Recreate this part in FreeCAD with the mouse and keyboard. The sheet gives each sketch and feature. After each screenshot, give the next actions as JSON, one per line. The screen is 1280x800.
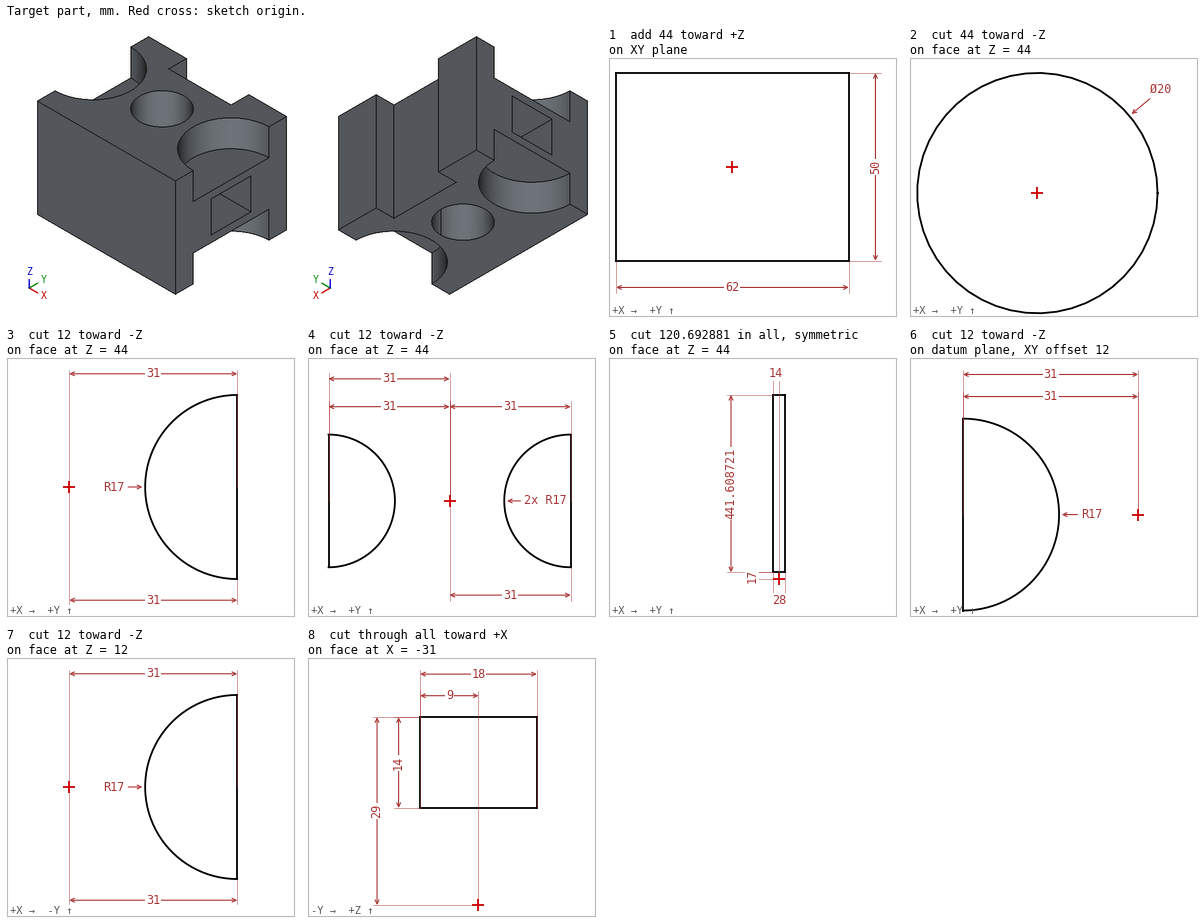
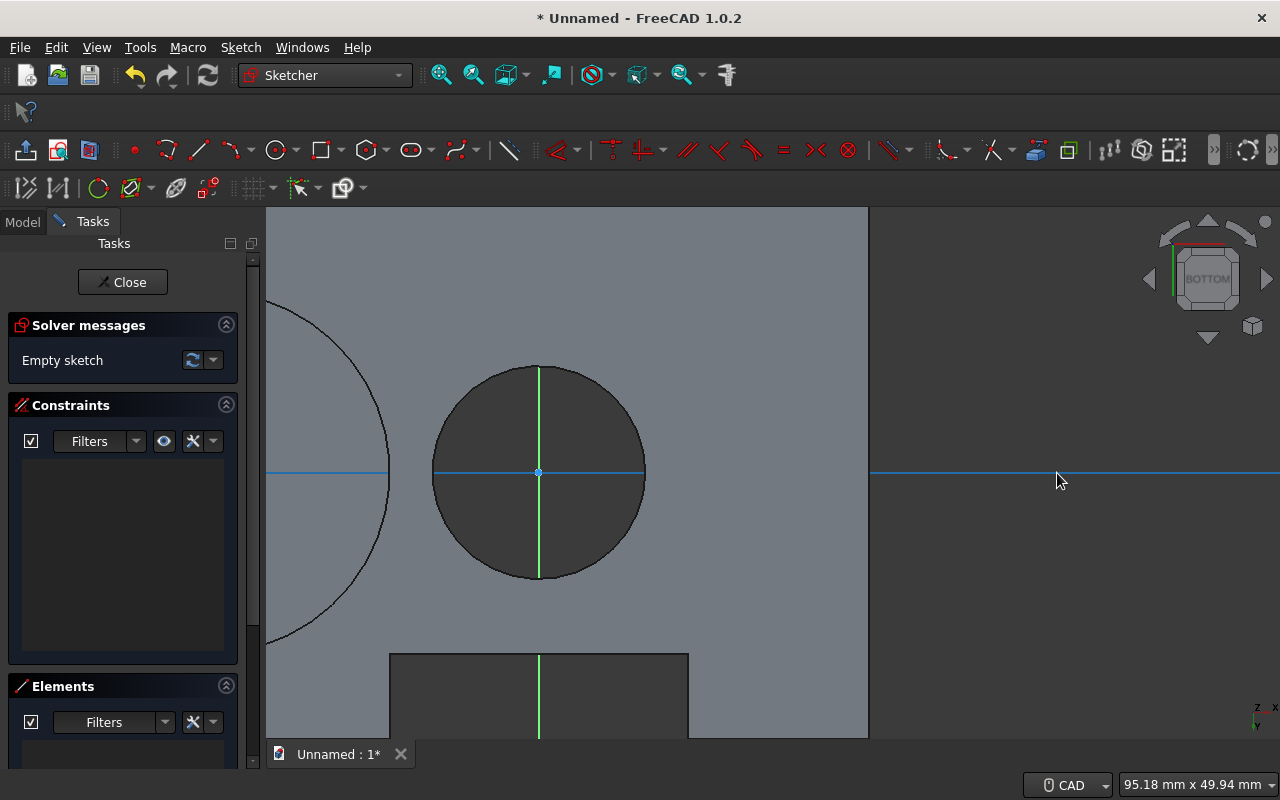
{"action": "left_click", "coordinate": [200, 150]}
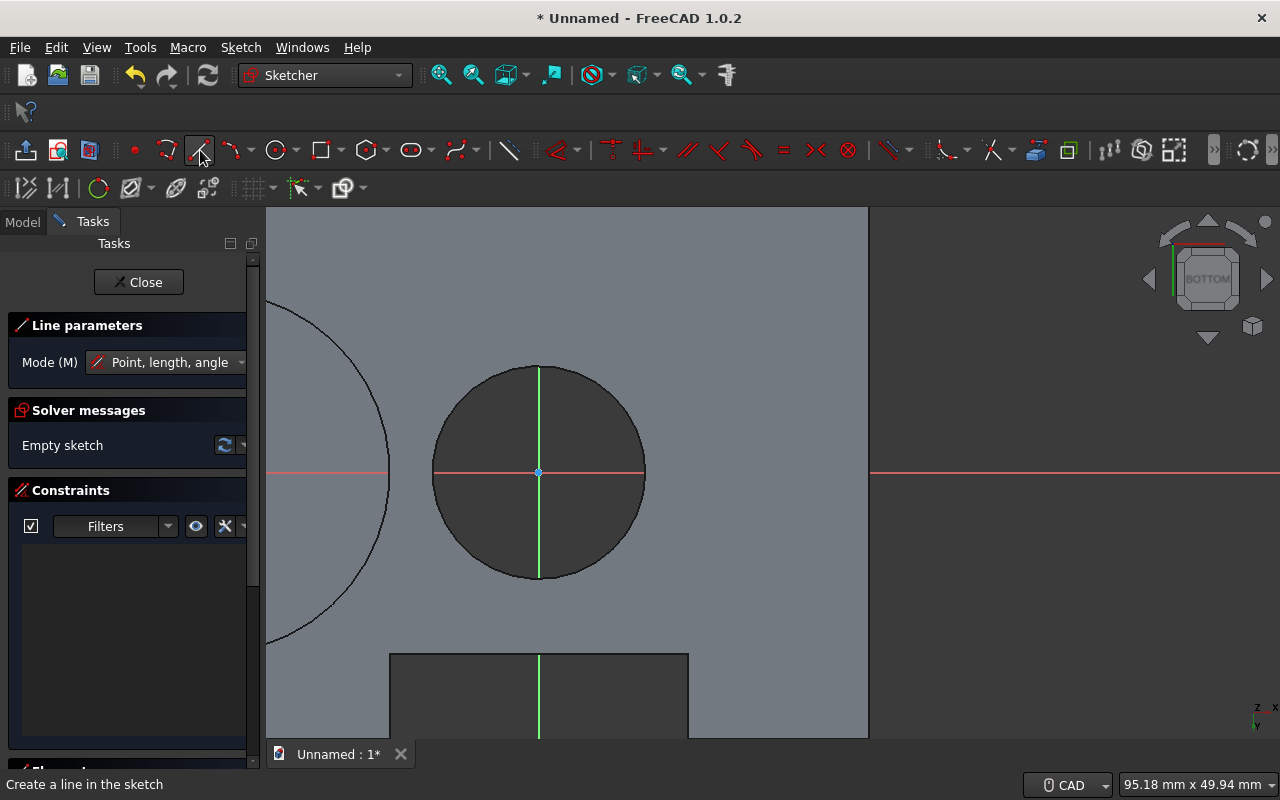
{"action": "left_click", "coordinate": [869, 654]}
{"action": "left_click", "coordinate": [869, 291]}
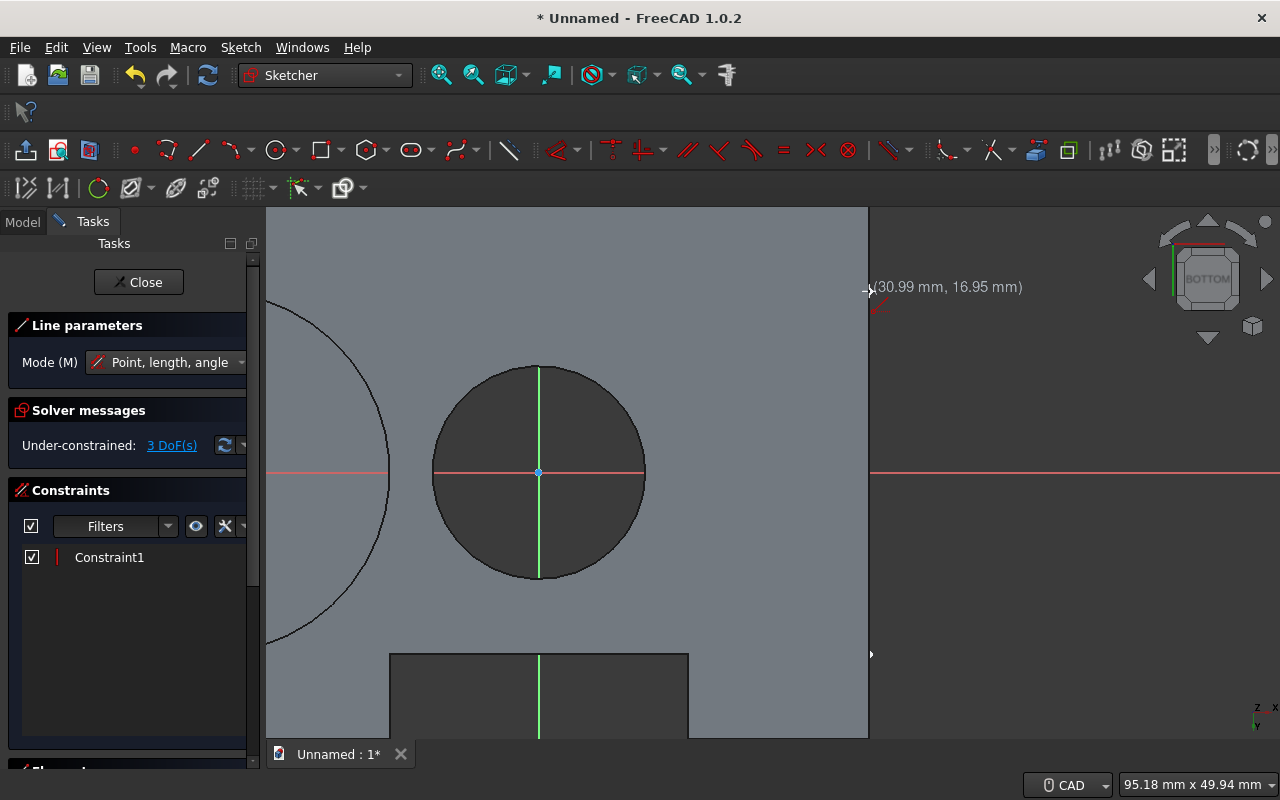
{"action": "key", "text": "g 3 a"}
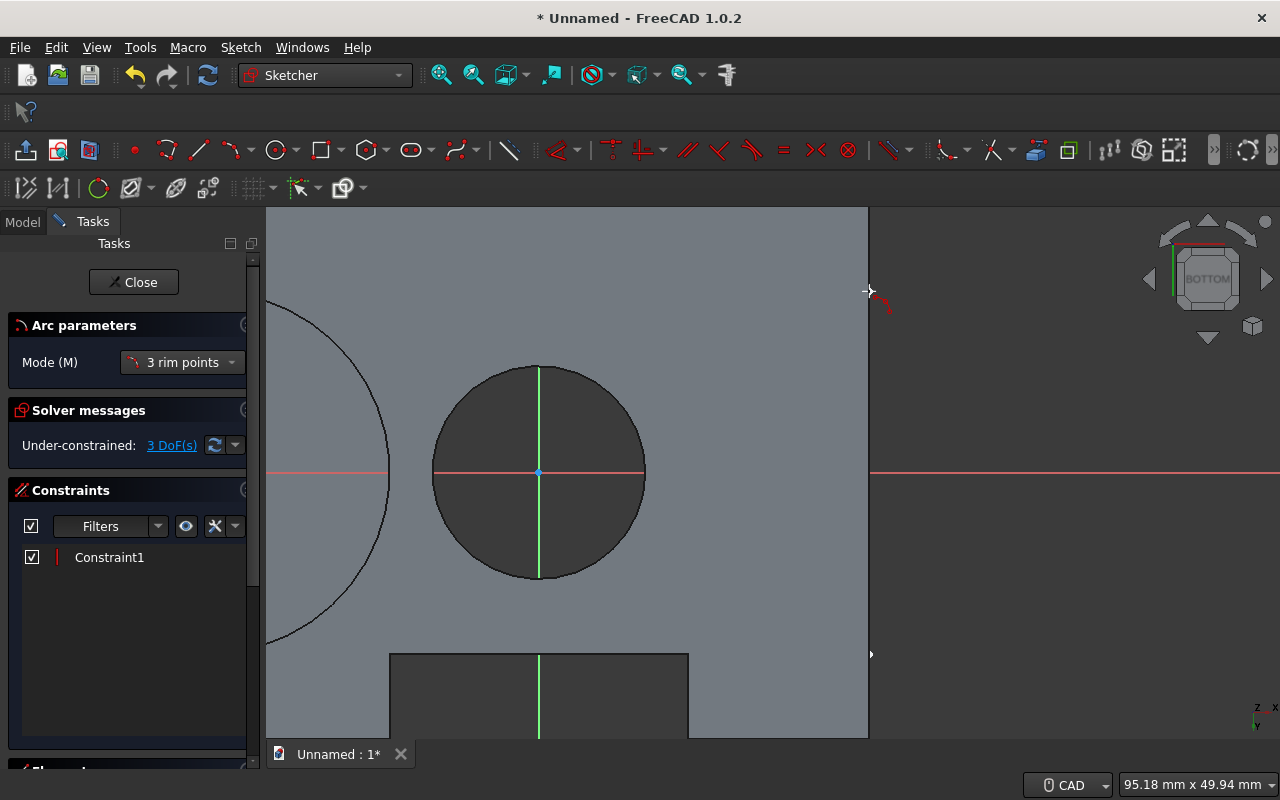
{"action": "left_click", "coordinate": [869, 292]}
{"action": "left_click", "coordinate": [869, 655]}
{"action": "left_click", "coordinate": [697, 417]}
{"action": "key", "text": "Escape"}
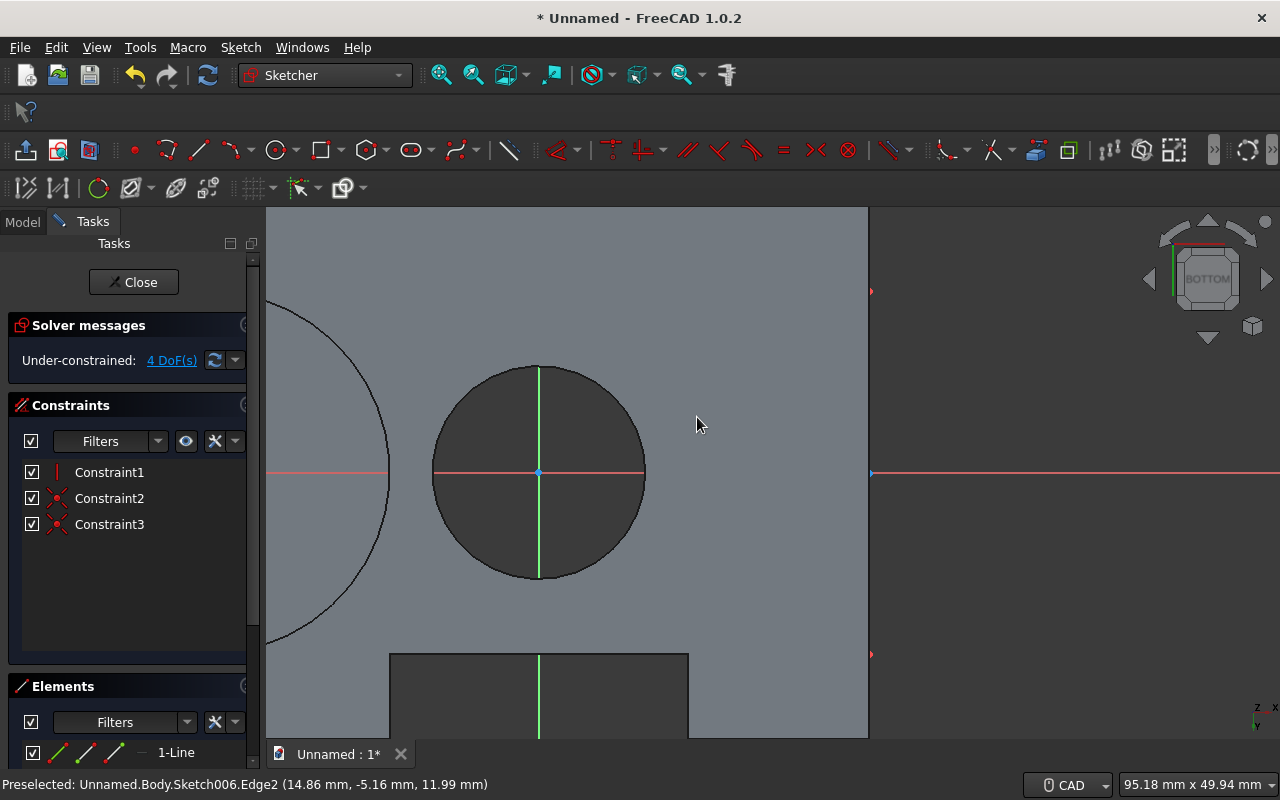
{"action": "left_click", "coordinate": [870, 473]}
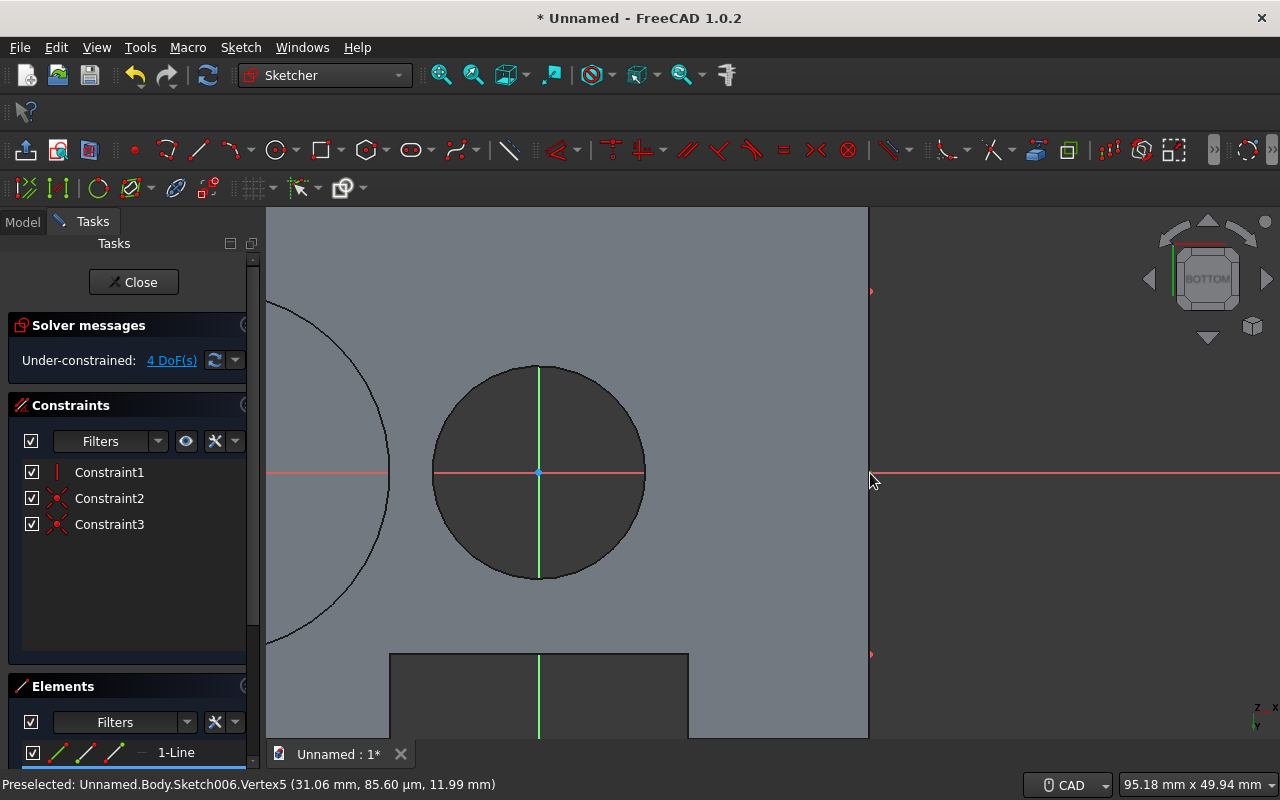
{"action": "left_click", "coordinate": [353, 473]}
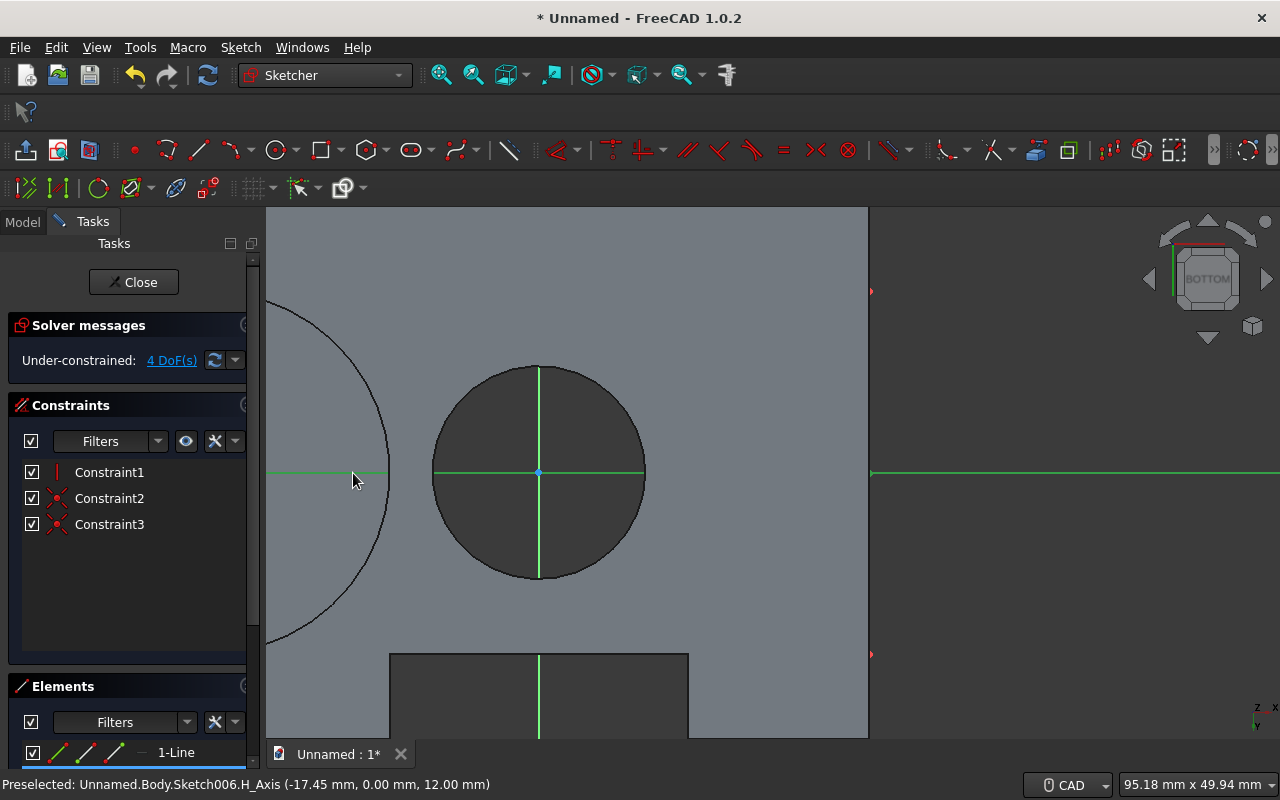
{"action": "key", "text": "c"}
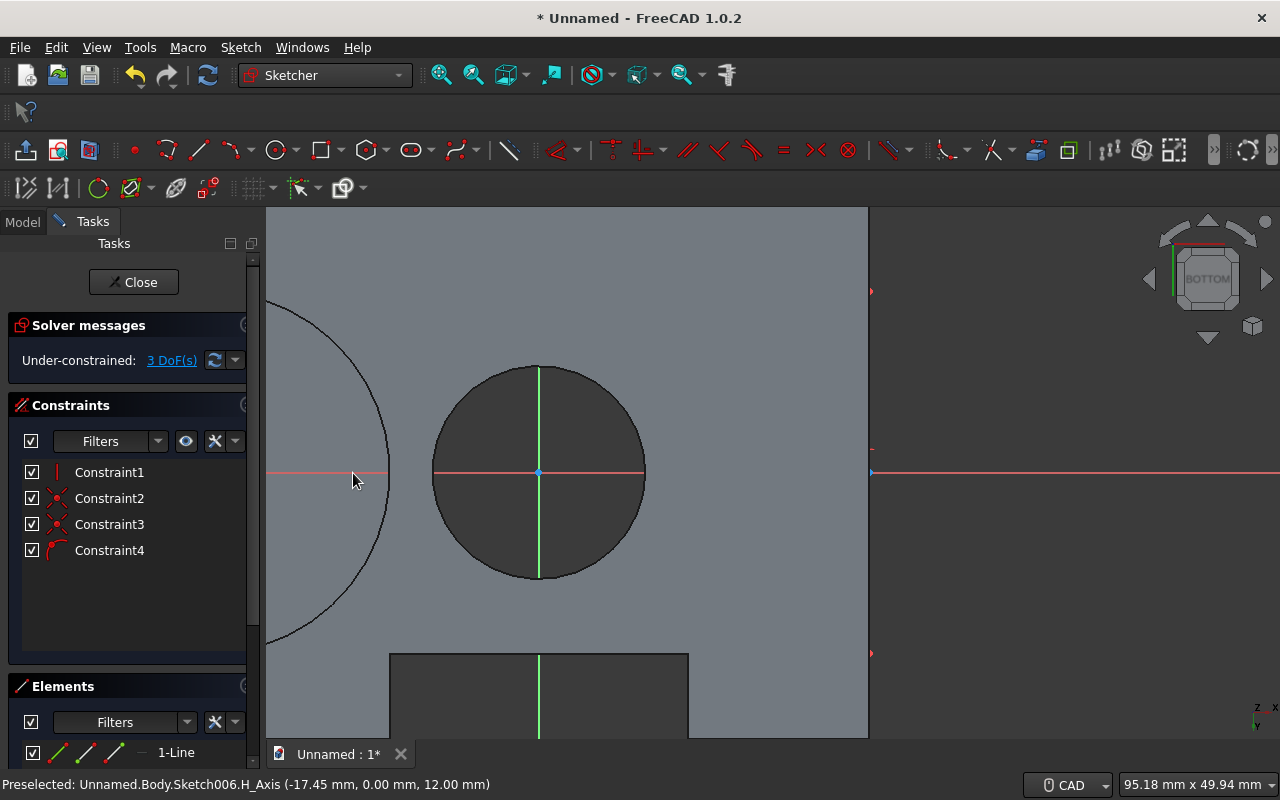
{"action": "left_click", "coordinate": [556, 150]}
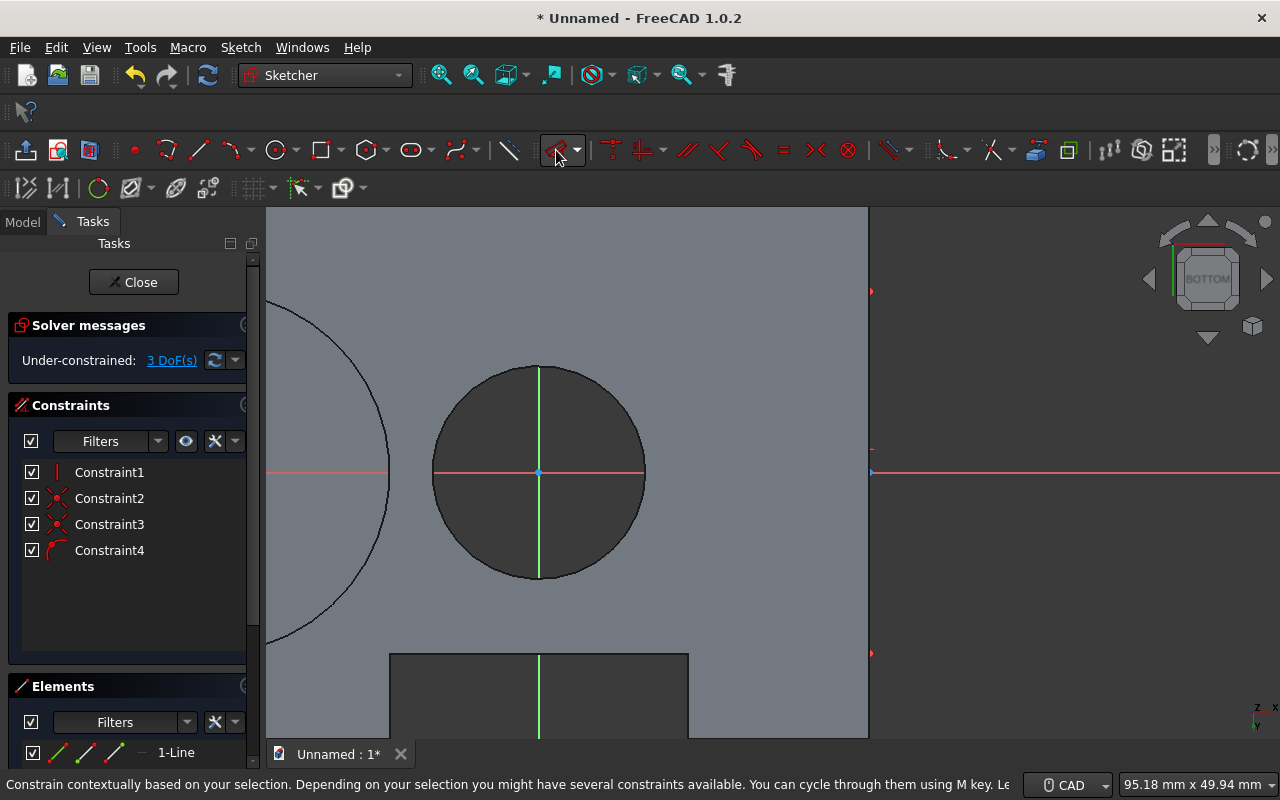
{"action": "left_click", "coordinate": [723, 366]}
{"action": "left_click", "coordinate": [697, 347]}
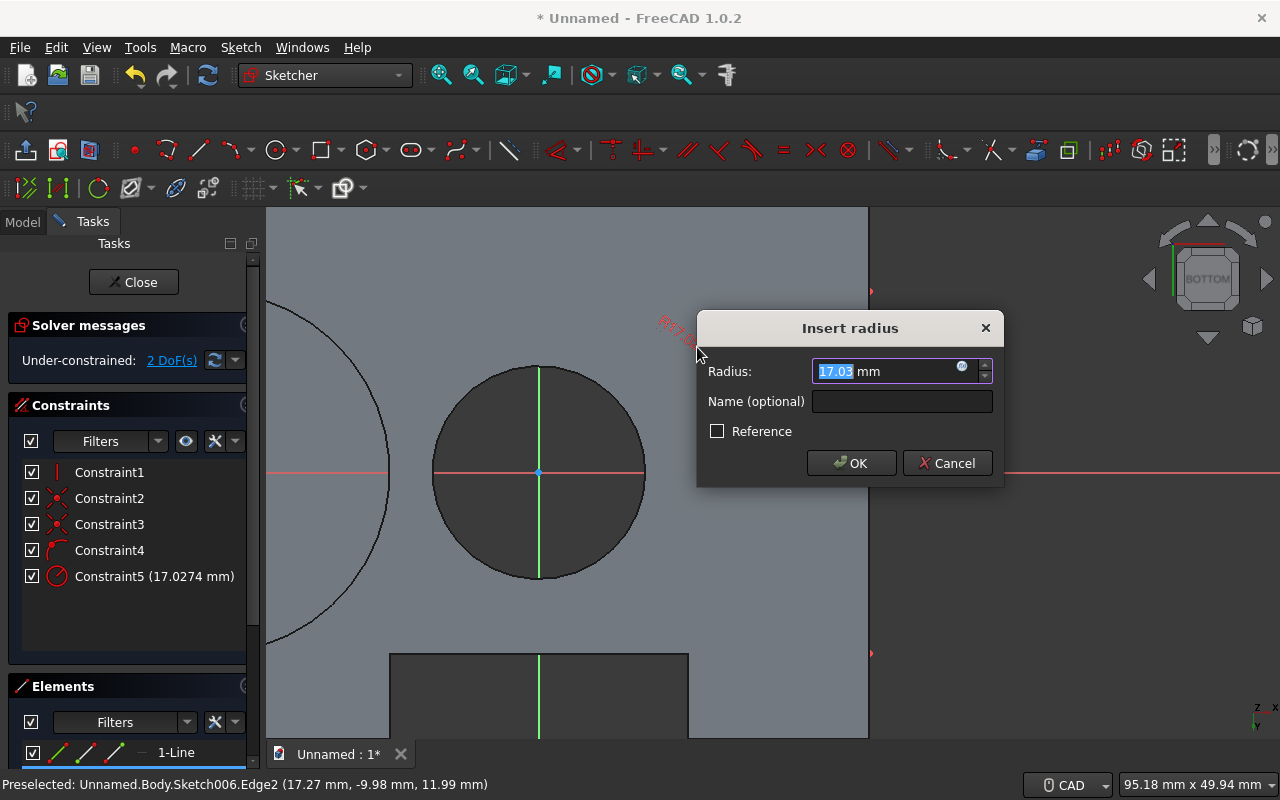
{"action": "type", "text": "17"}
{"action": "key", "text": "Return"}